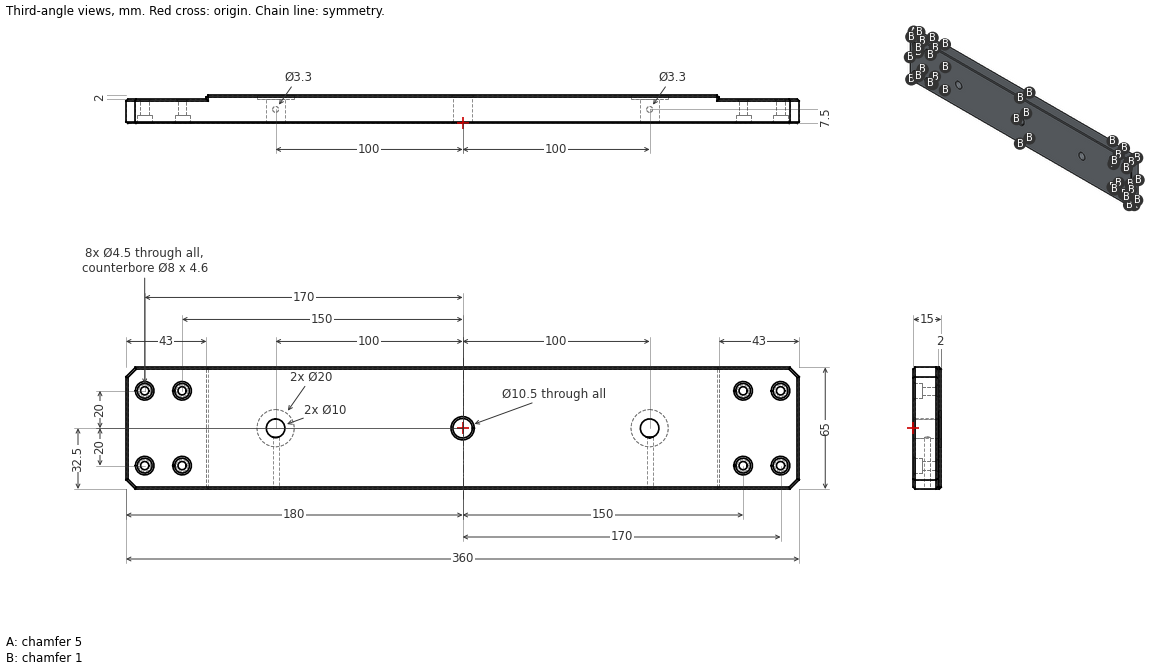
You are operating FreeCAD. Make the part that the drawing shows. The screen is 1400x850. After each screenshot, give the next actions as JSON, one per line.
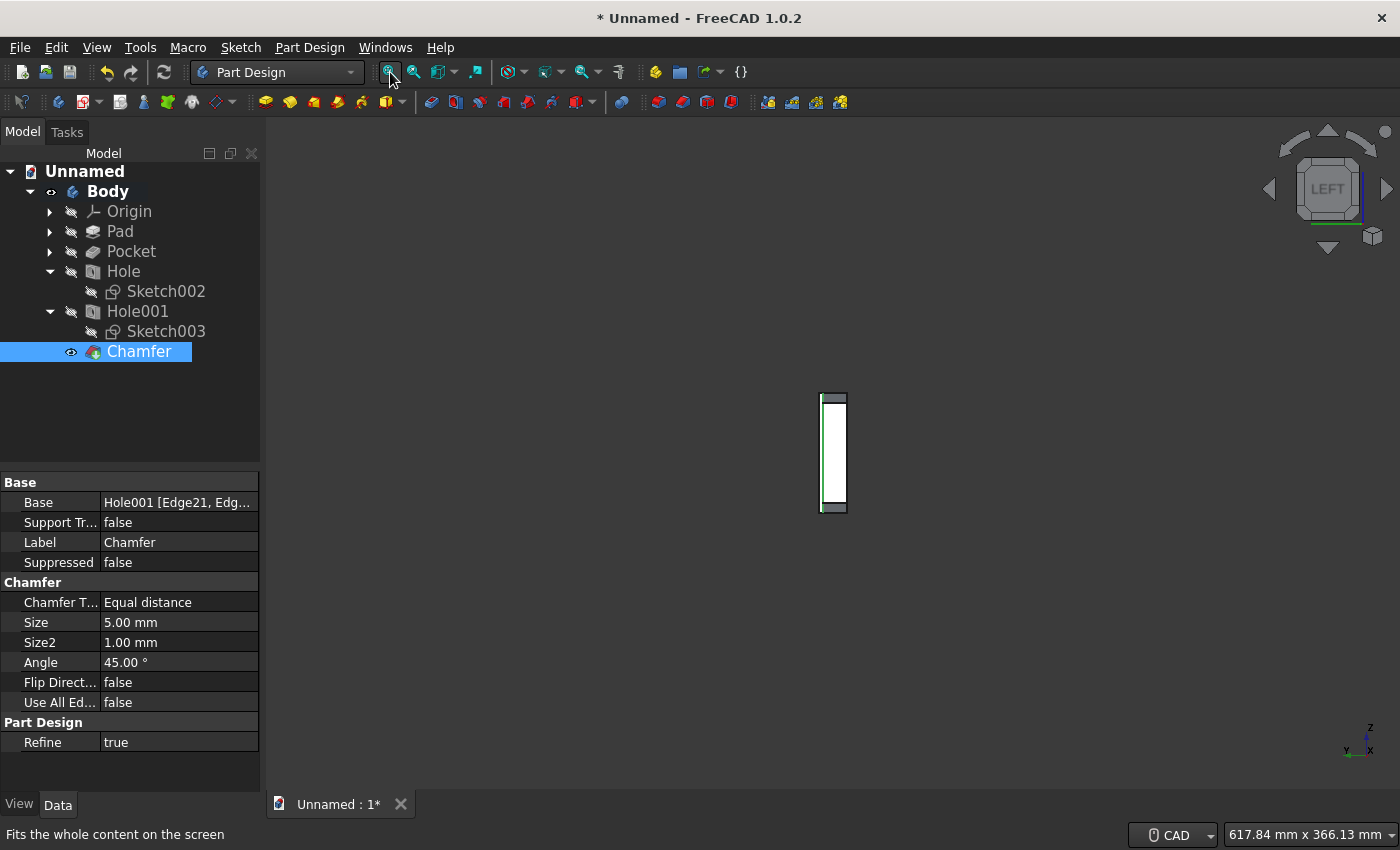
{"action": "left_click", "coordinate": [390, 72]}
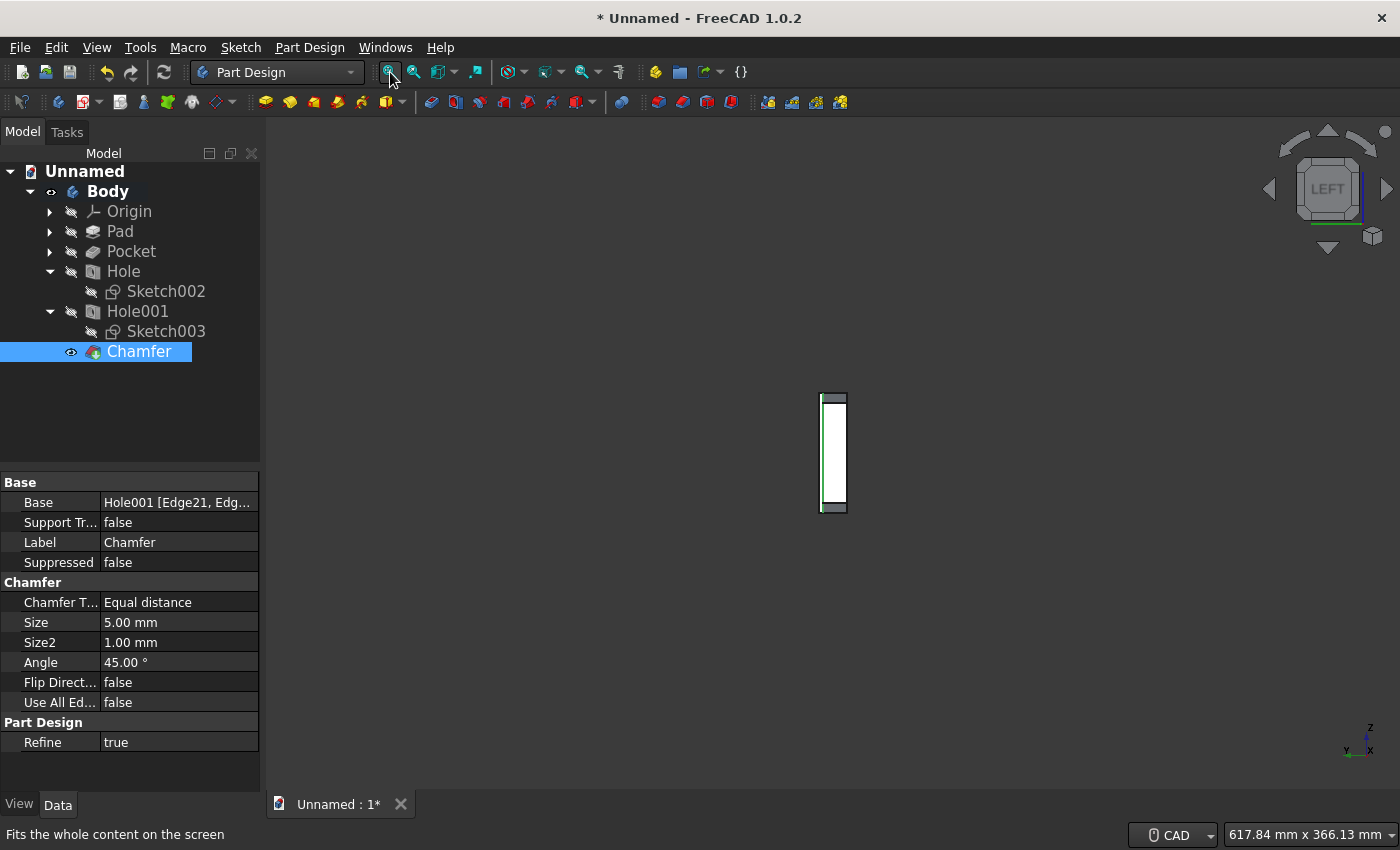
{"action": "scroll", "coordinate": [821, 512], "scroll_direction": "up", "scroll_amount": 12}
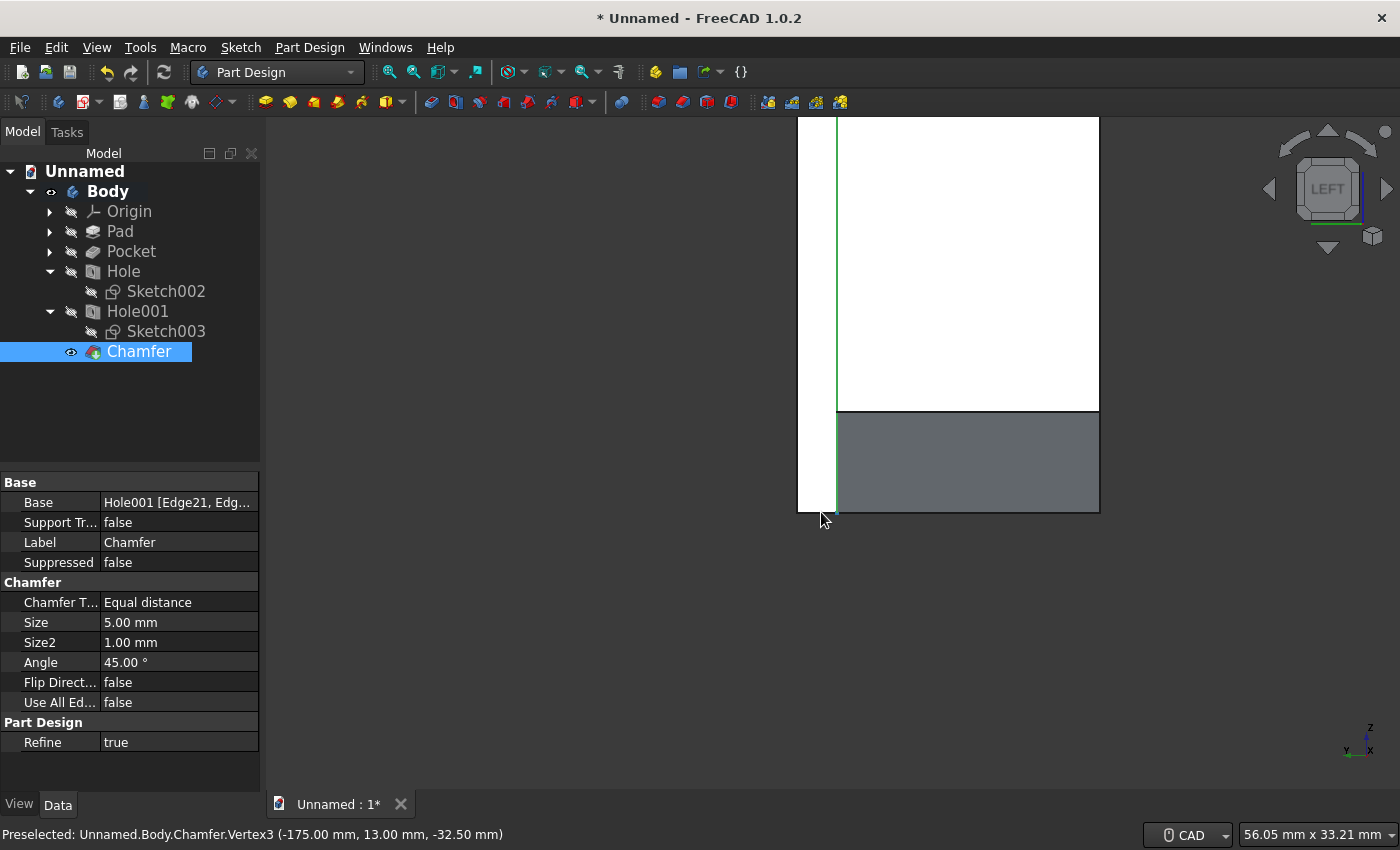
{"action": "left_click", "coordinate": [817, 512], "text": "ctrl"}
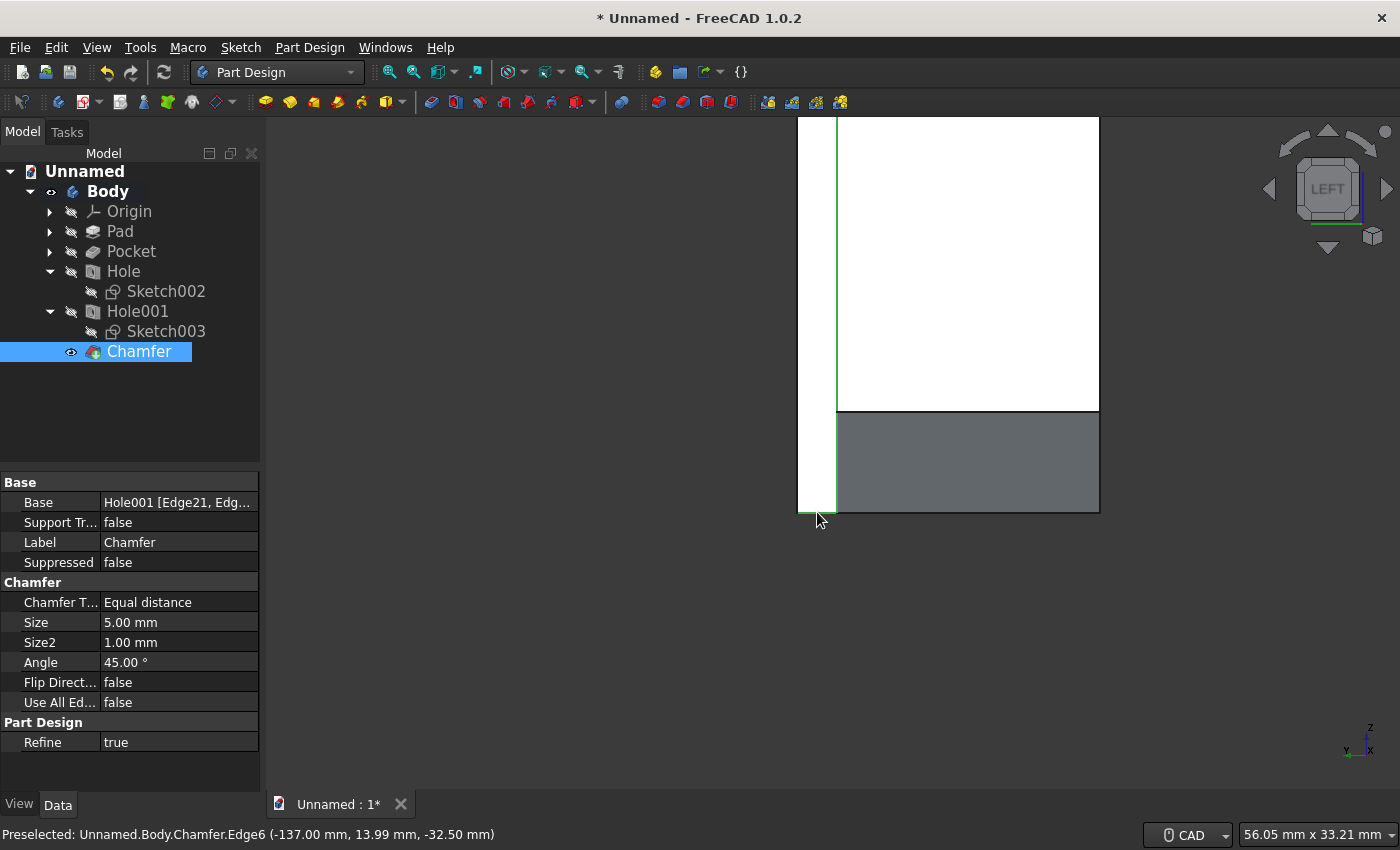
{"action": "left_click", "coordinate": [390, 72]}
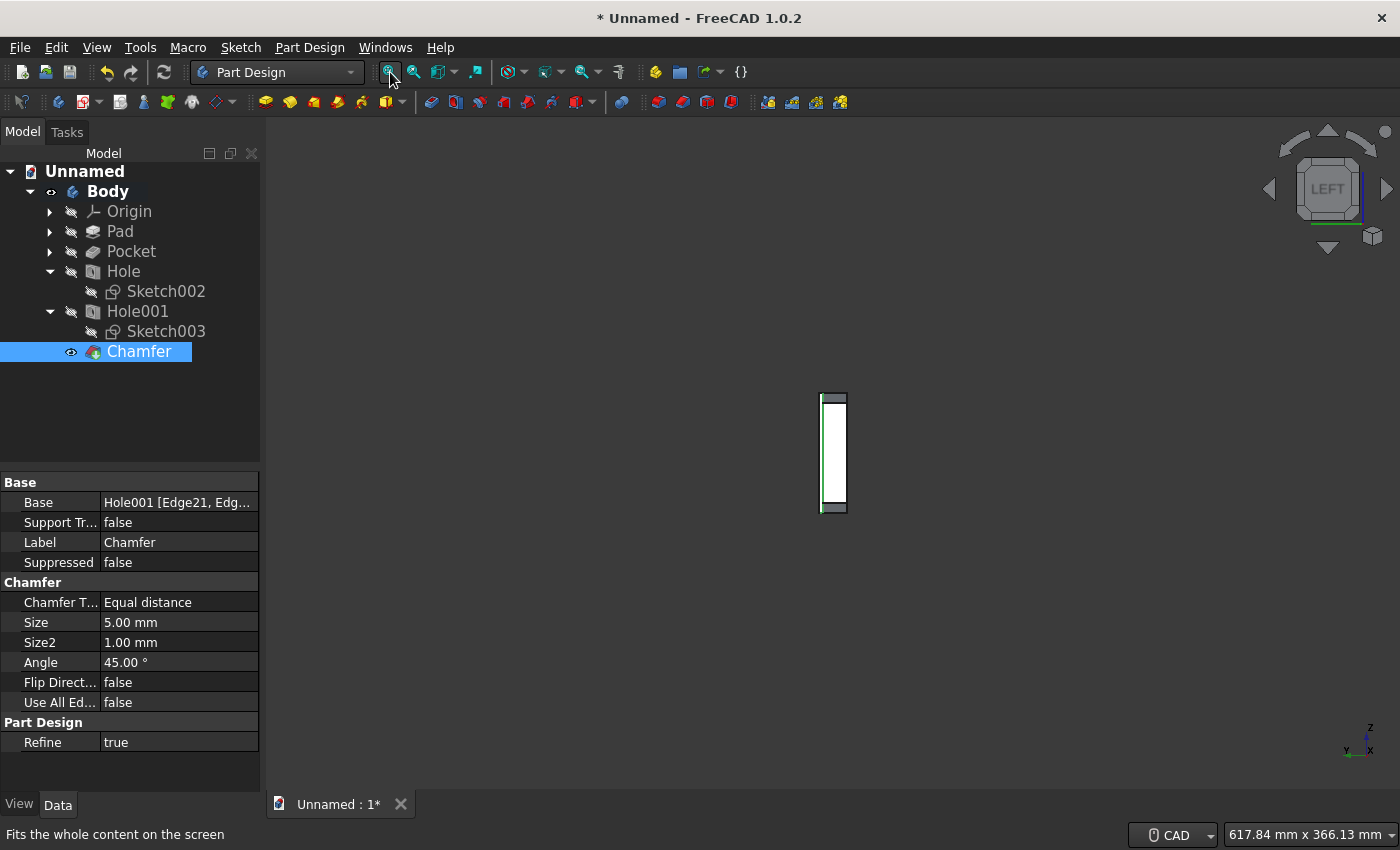
{"action": "key", "text": "v 3"}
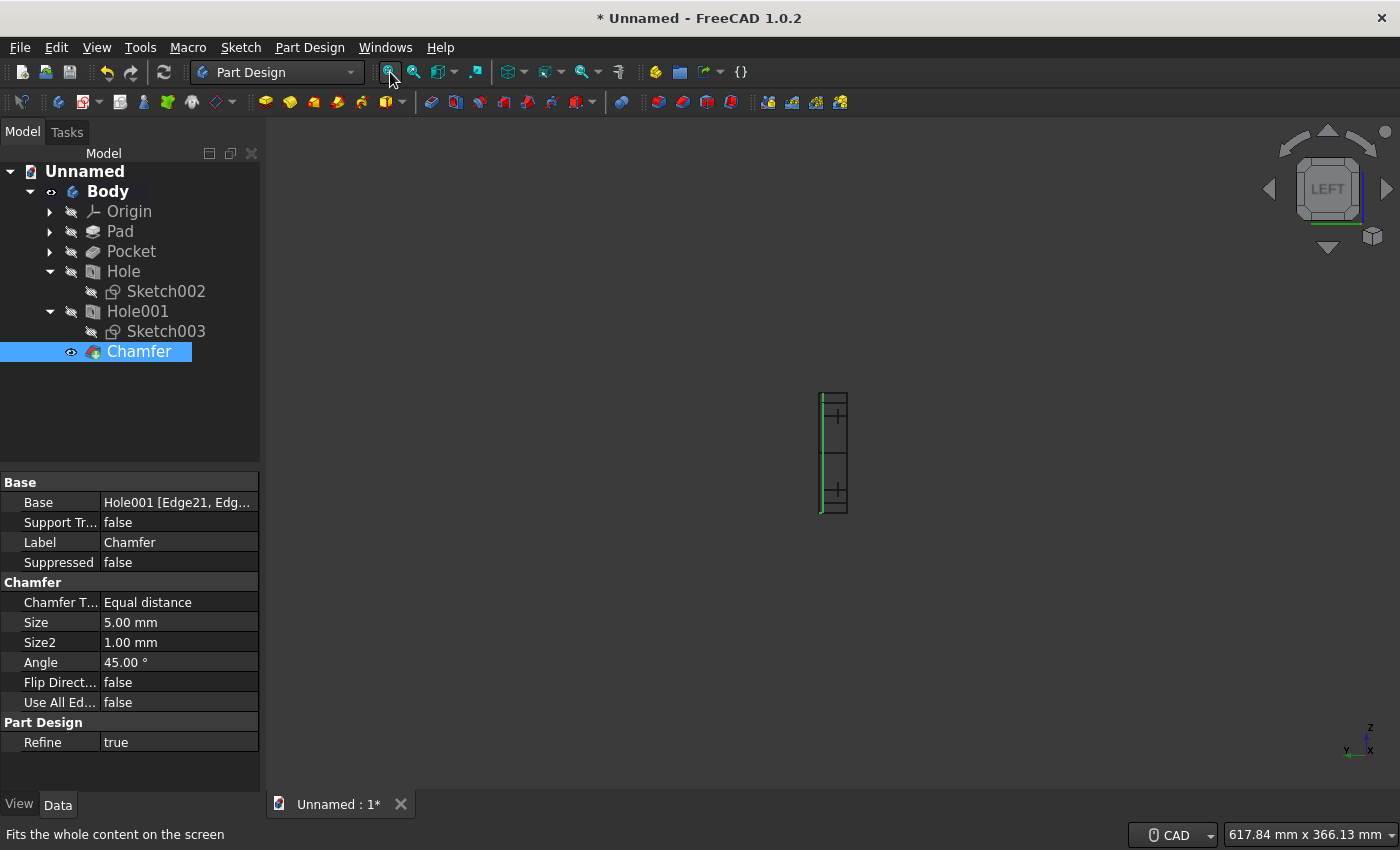
{"action": "key", "text": "0"}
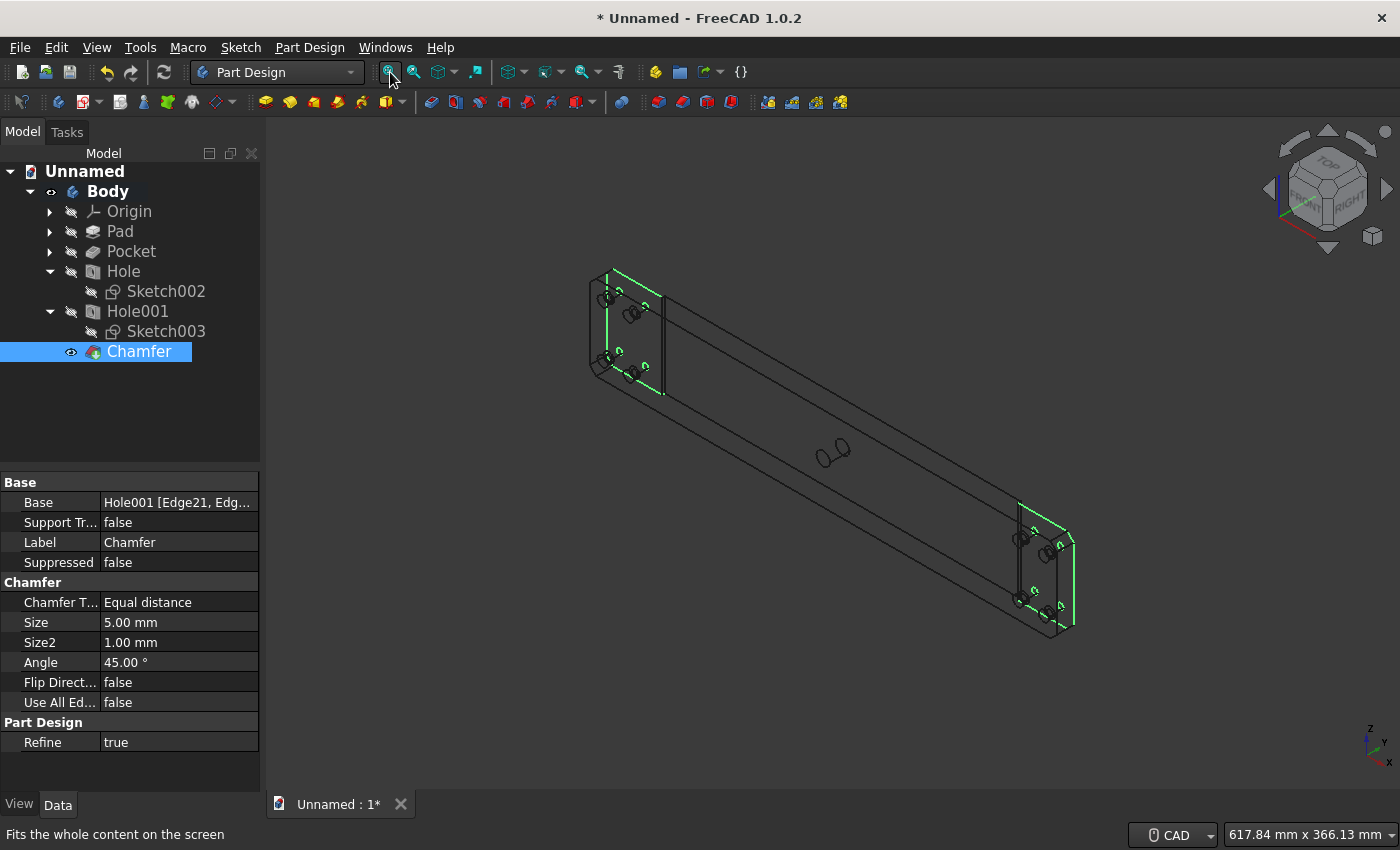
{"action": "scroll", "coordinate": [664, 296], "scroll_direction": "up", "scroll_amount": 12}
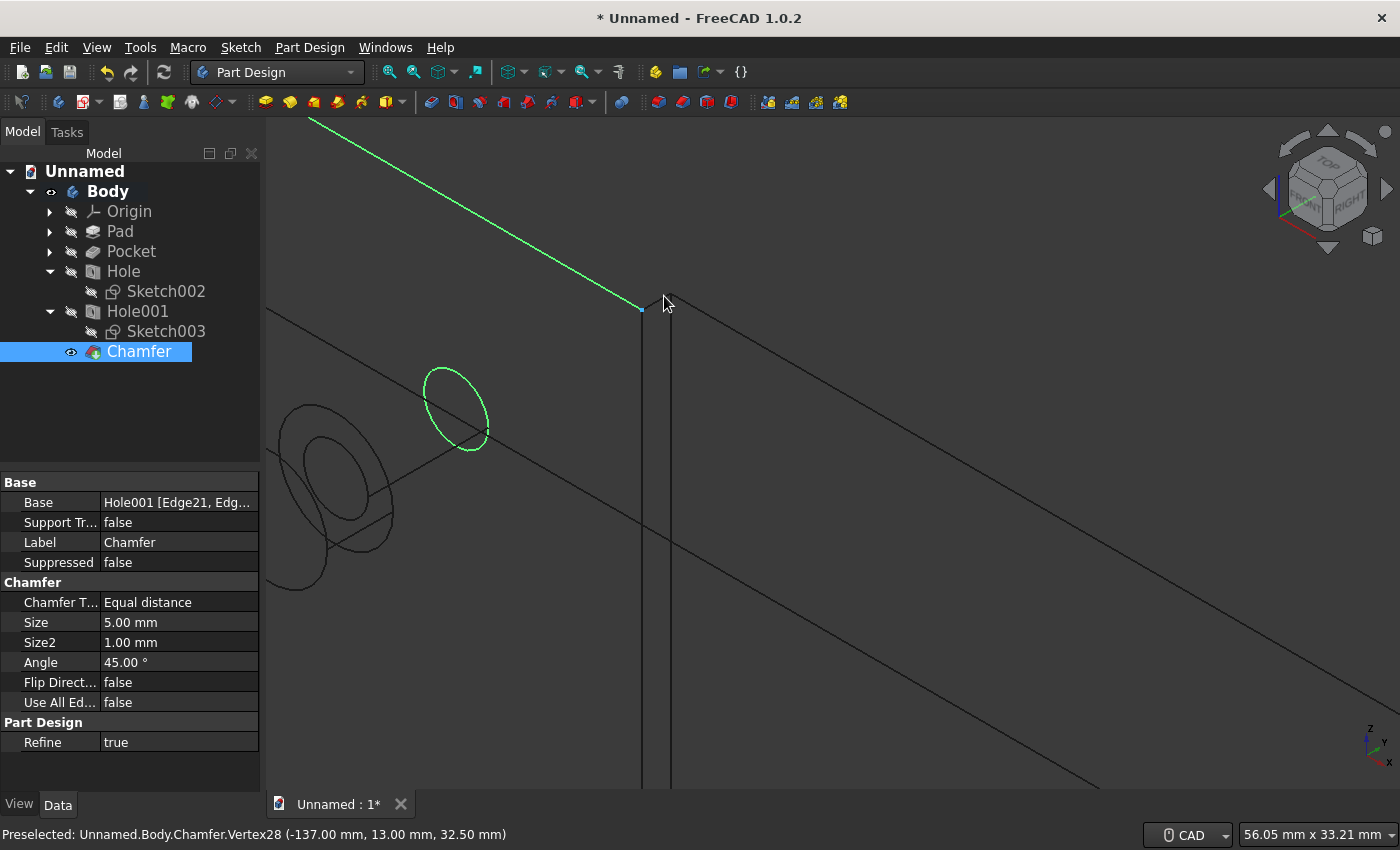
{"action": "left_click", "coordinate": [656, 301], "text": "ctrl"}